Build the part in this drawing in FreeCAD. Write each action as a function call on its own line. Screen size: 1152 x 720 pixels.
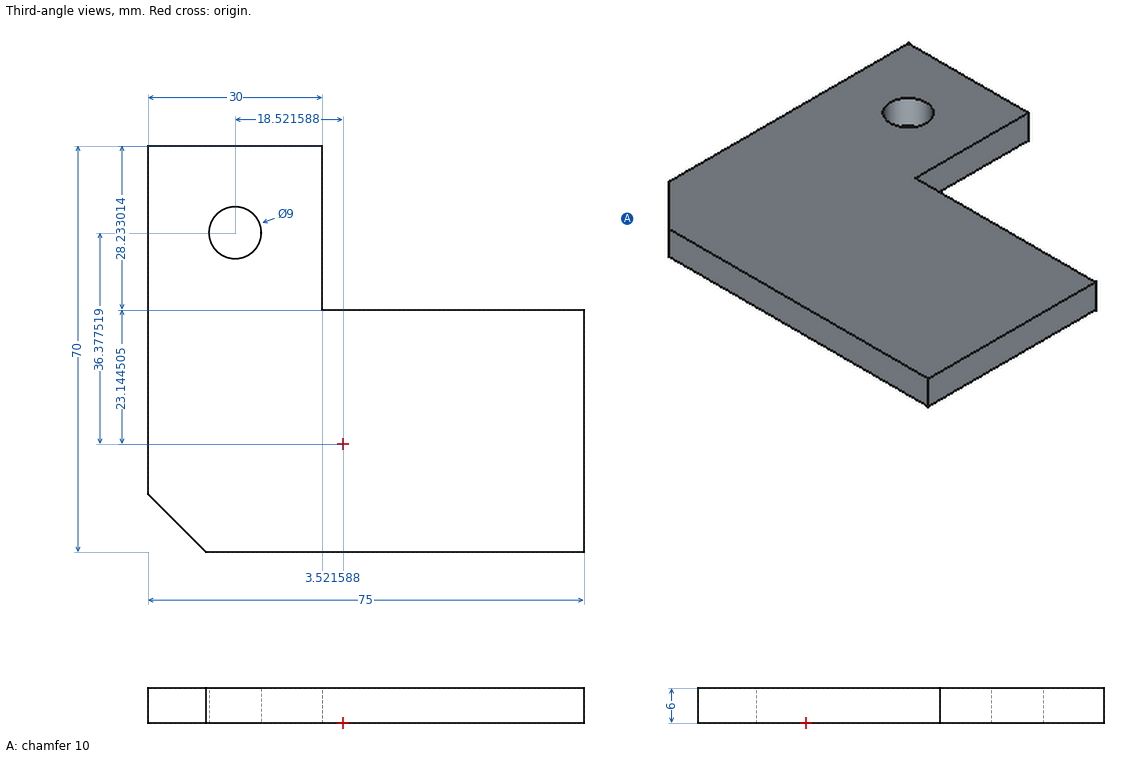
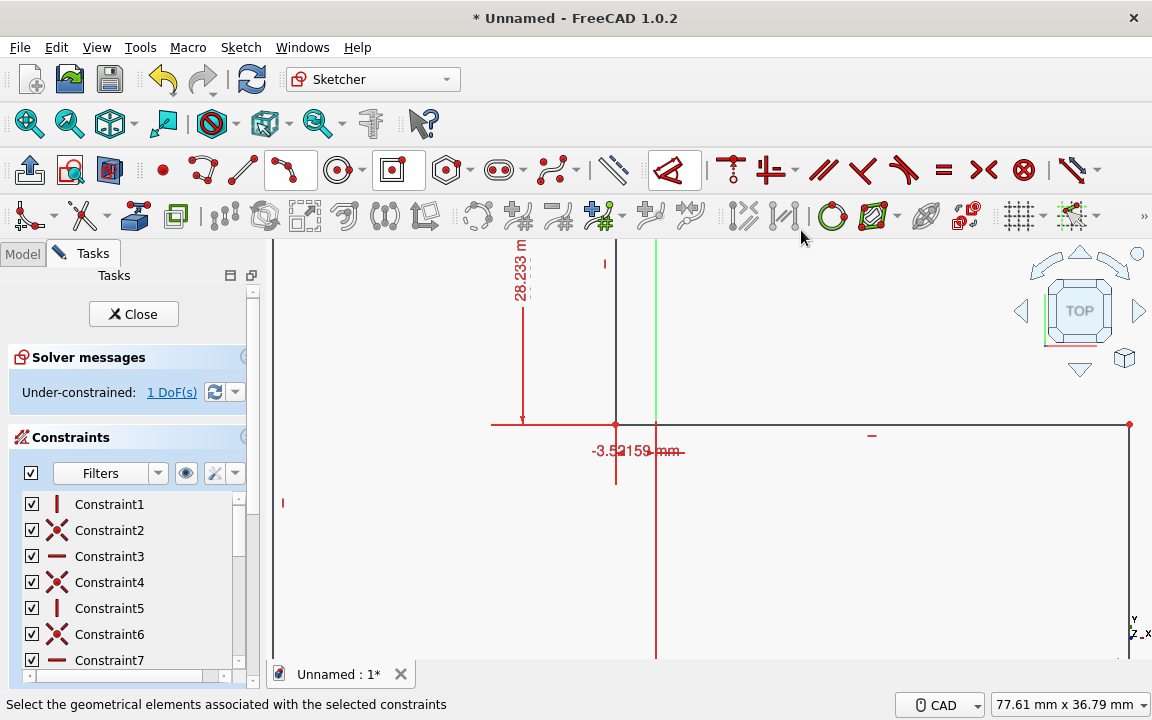
click(616, 425)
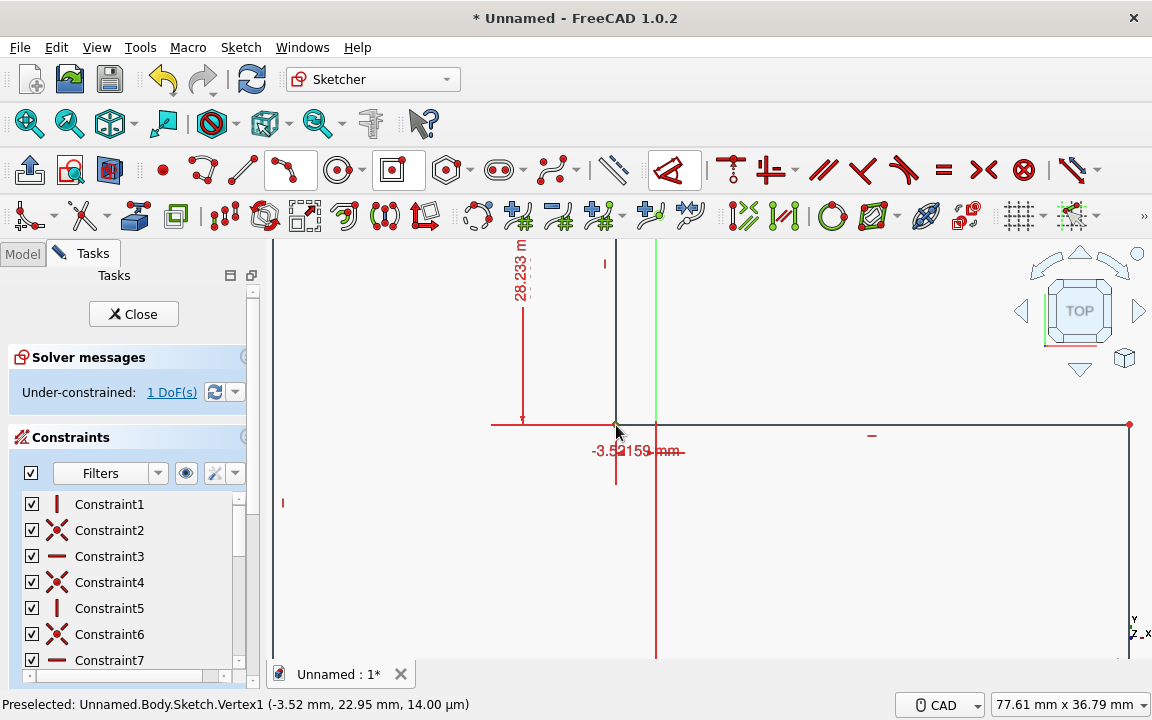
key(i)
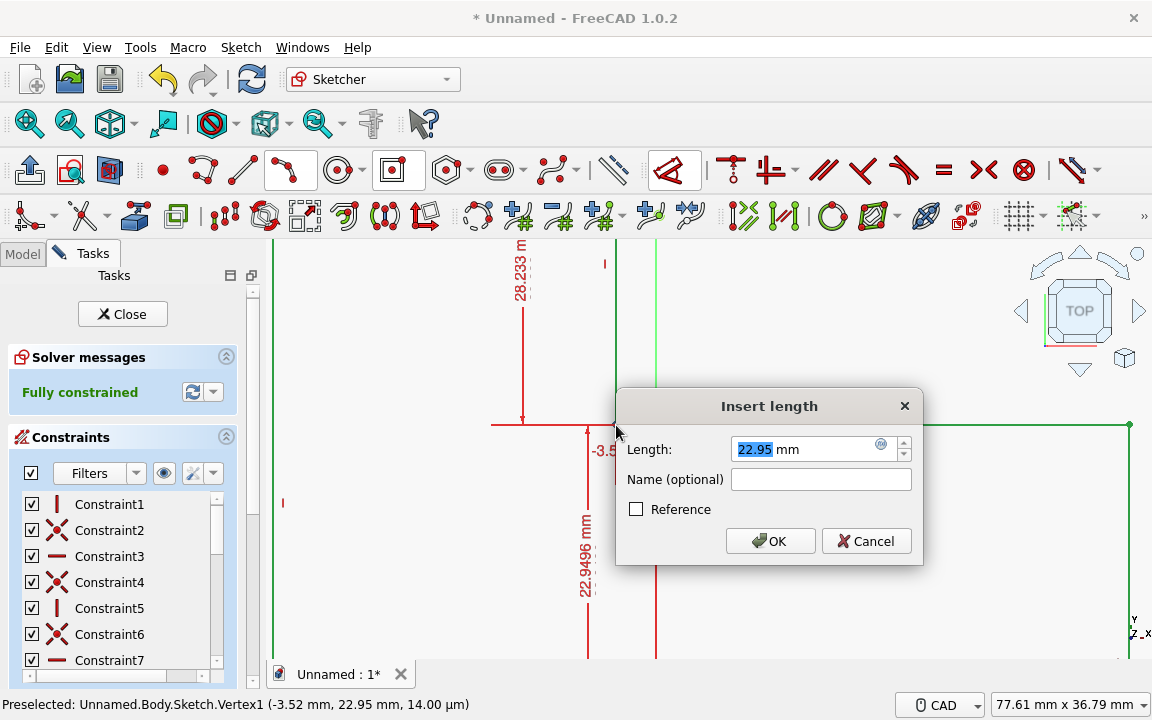
text(23.144505)
key(Return)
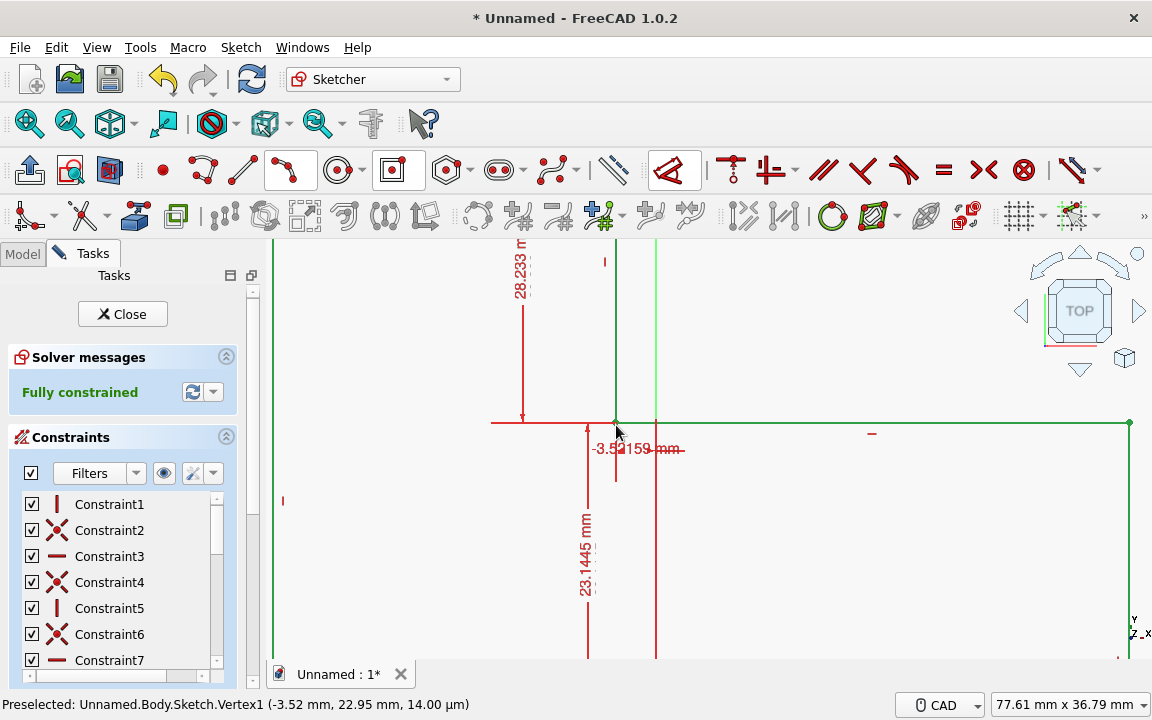
click(123, 314)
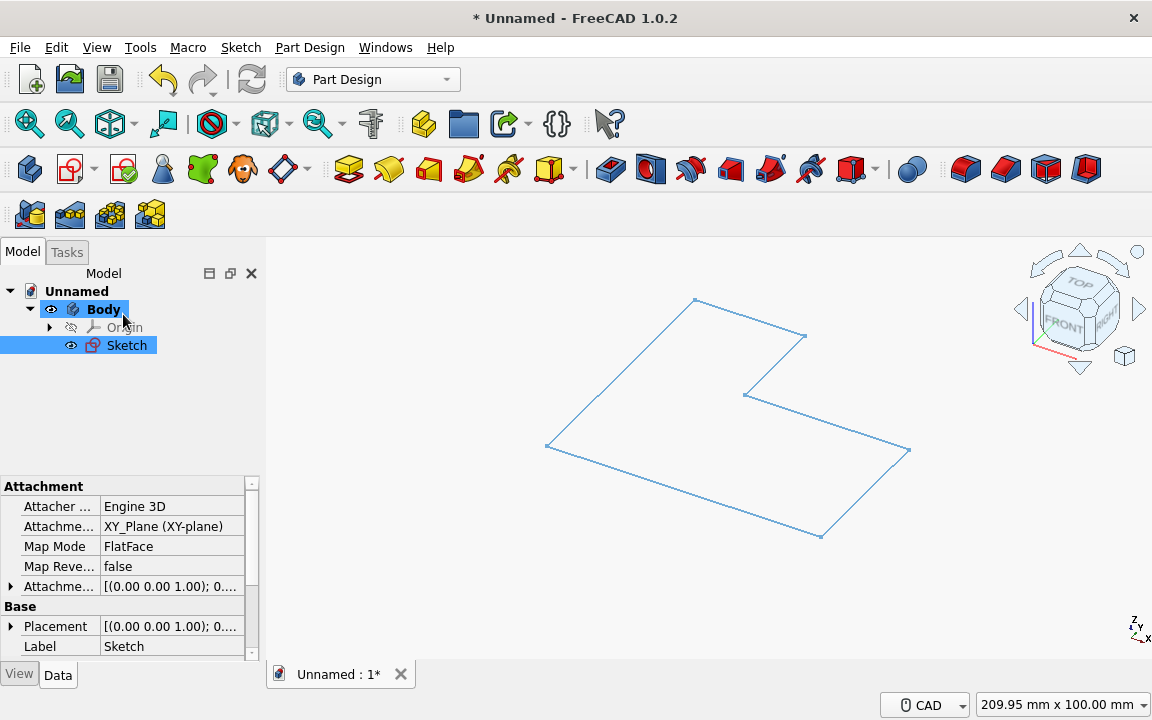
click(350, 170)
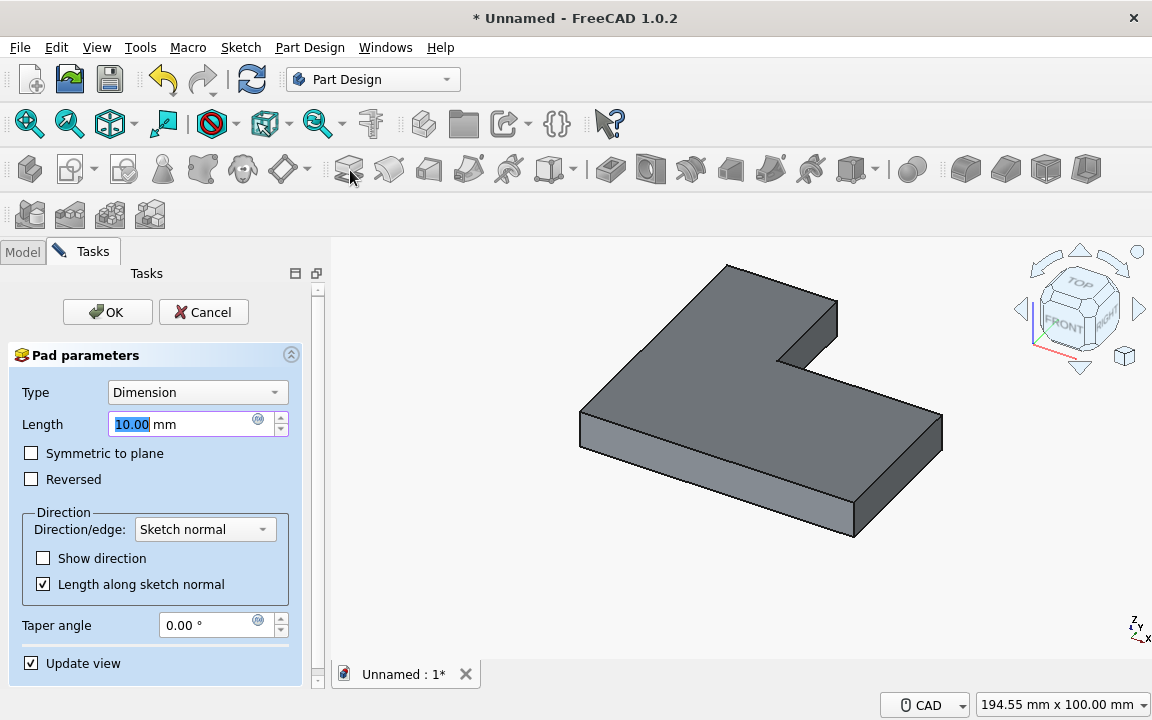
text(6)
key(Tab)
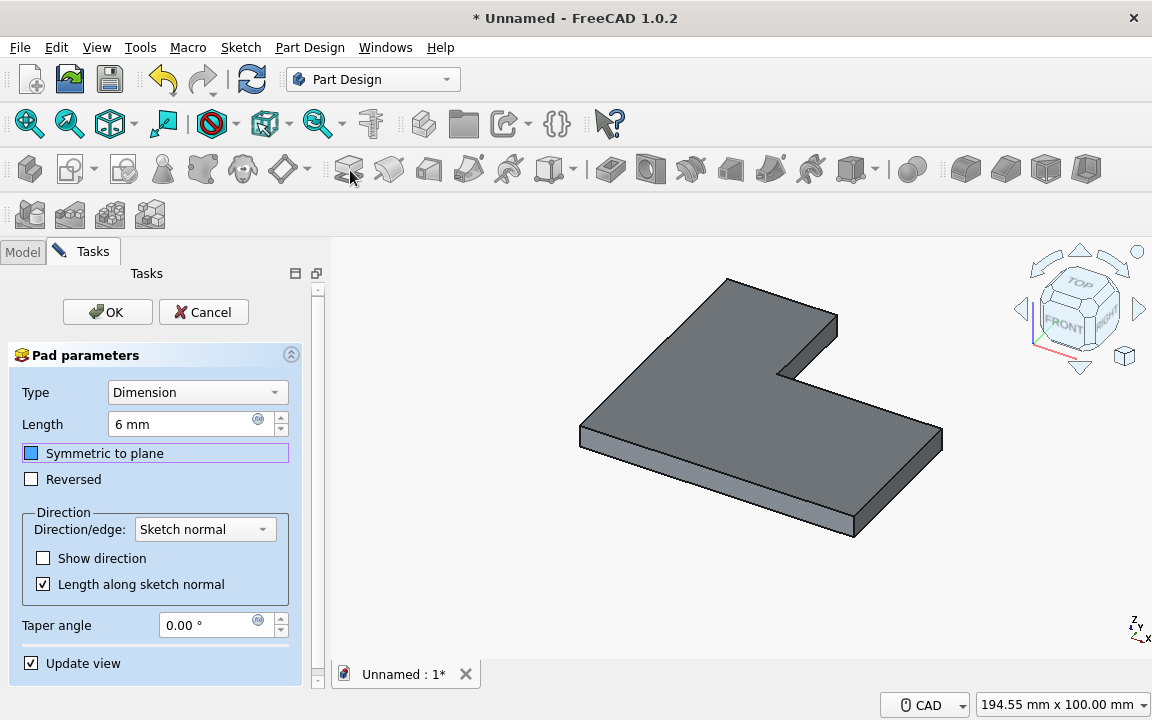
click(108, 312)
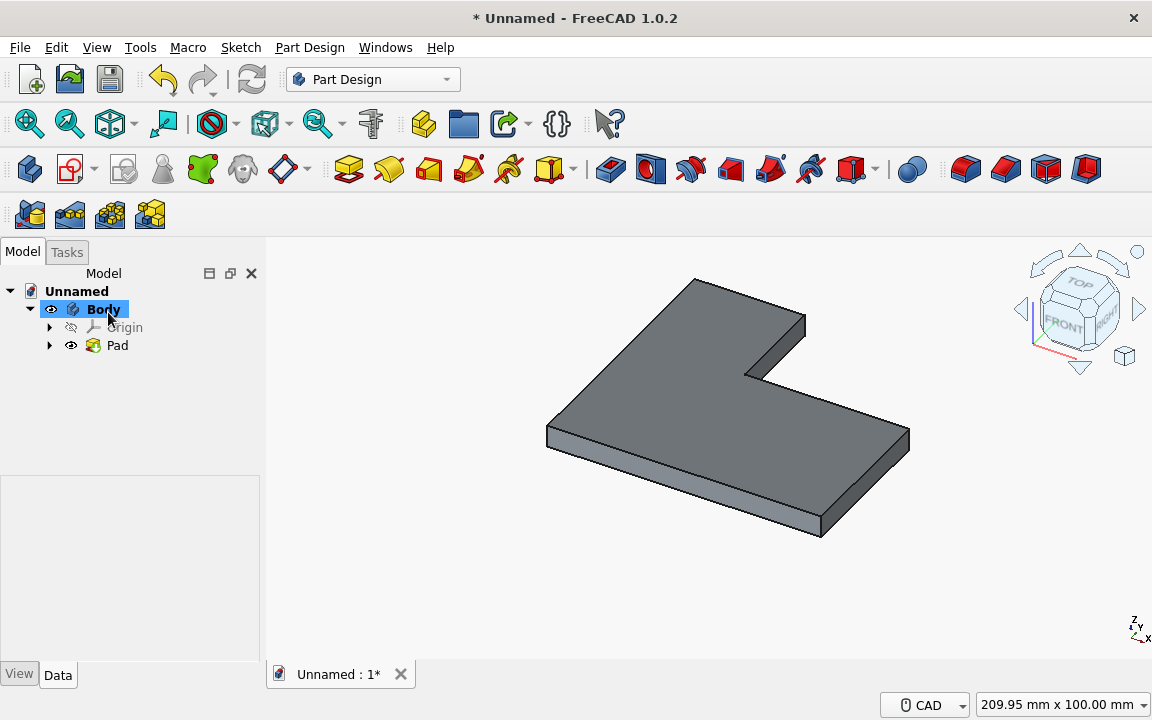
click(698, 405)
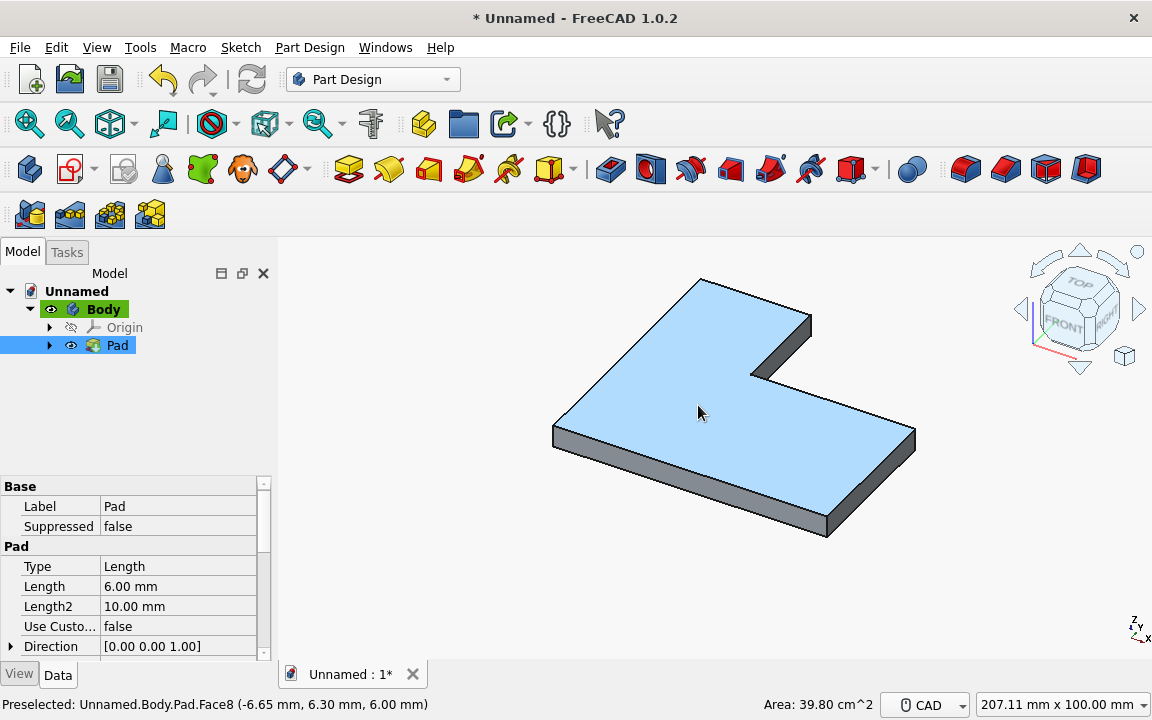
click(70, 170)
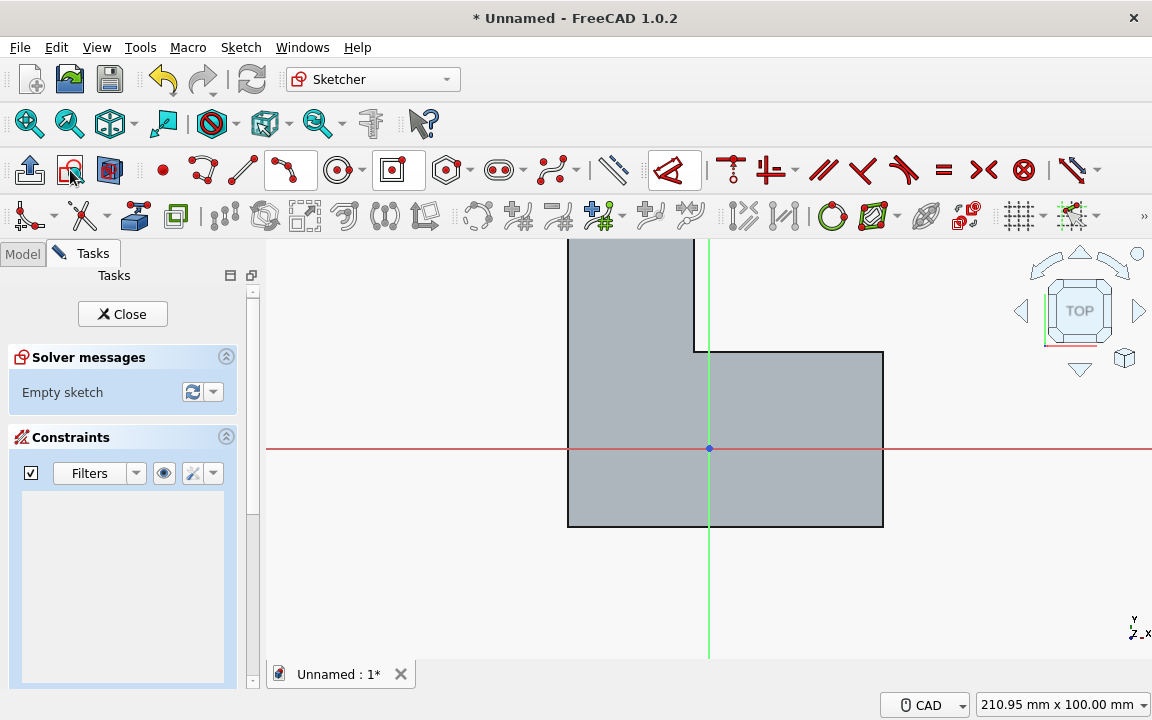
scroll(630, 272, up, 10)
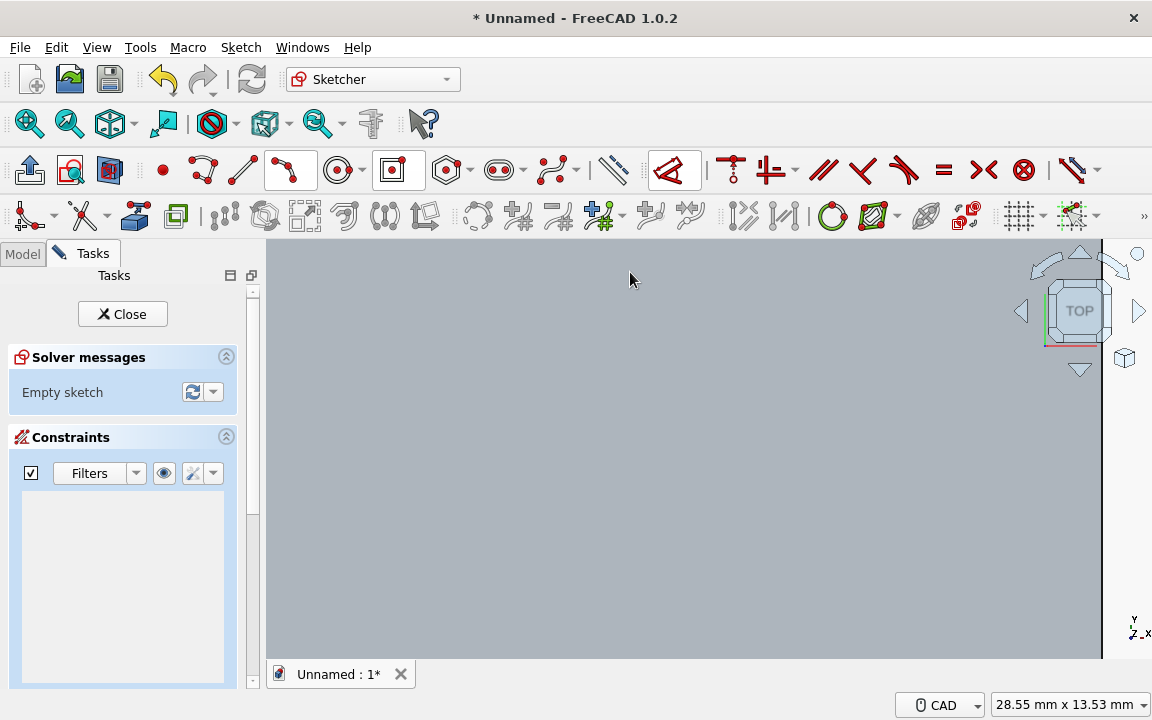
click(338, 170)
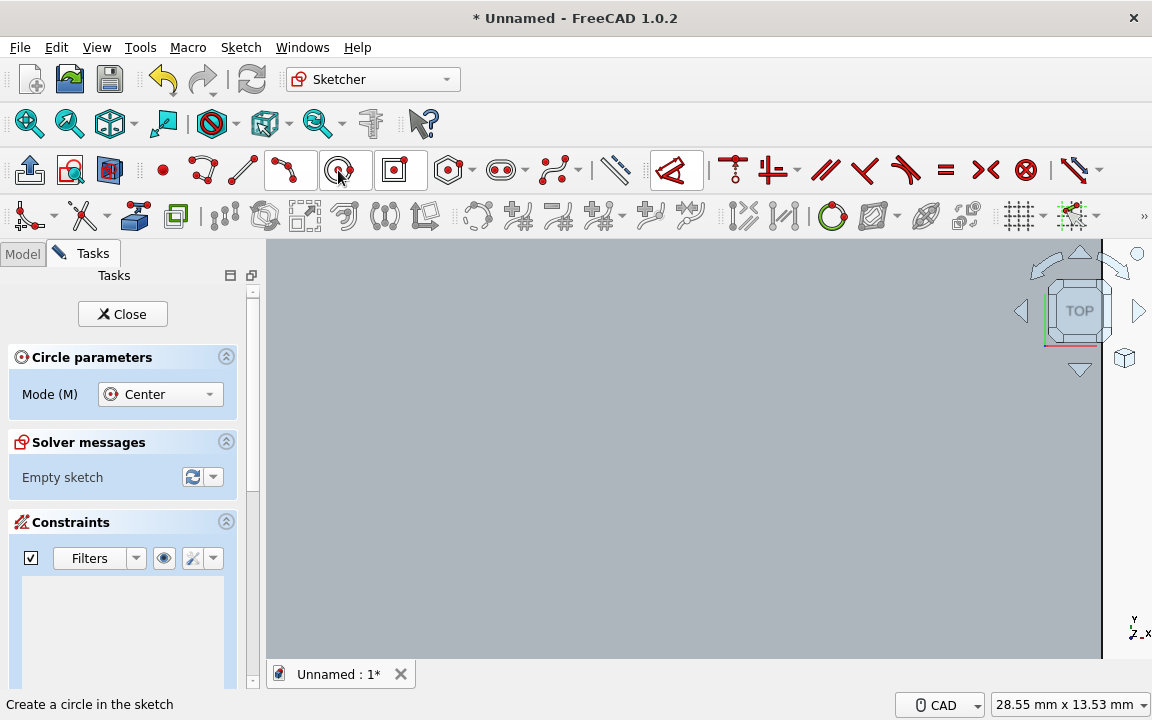
click(636, 450)
move(735, 352)